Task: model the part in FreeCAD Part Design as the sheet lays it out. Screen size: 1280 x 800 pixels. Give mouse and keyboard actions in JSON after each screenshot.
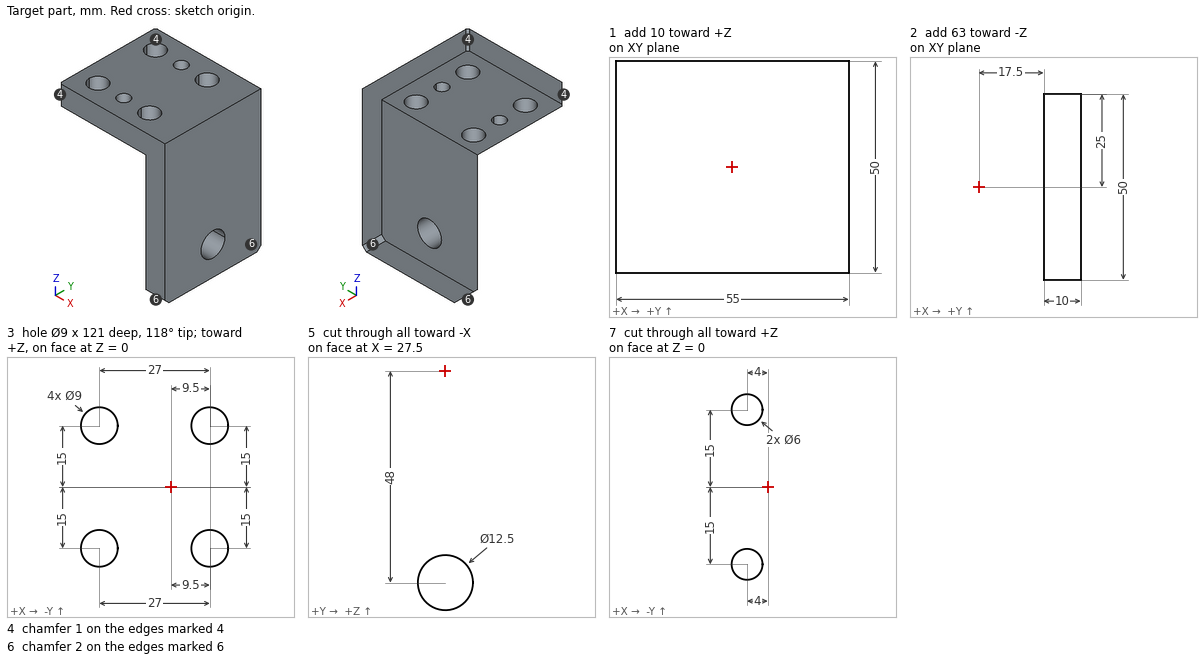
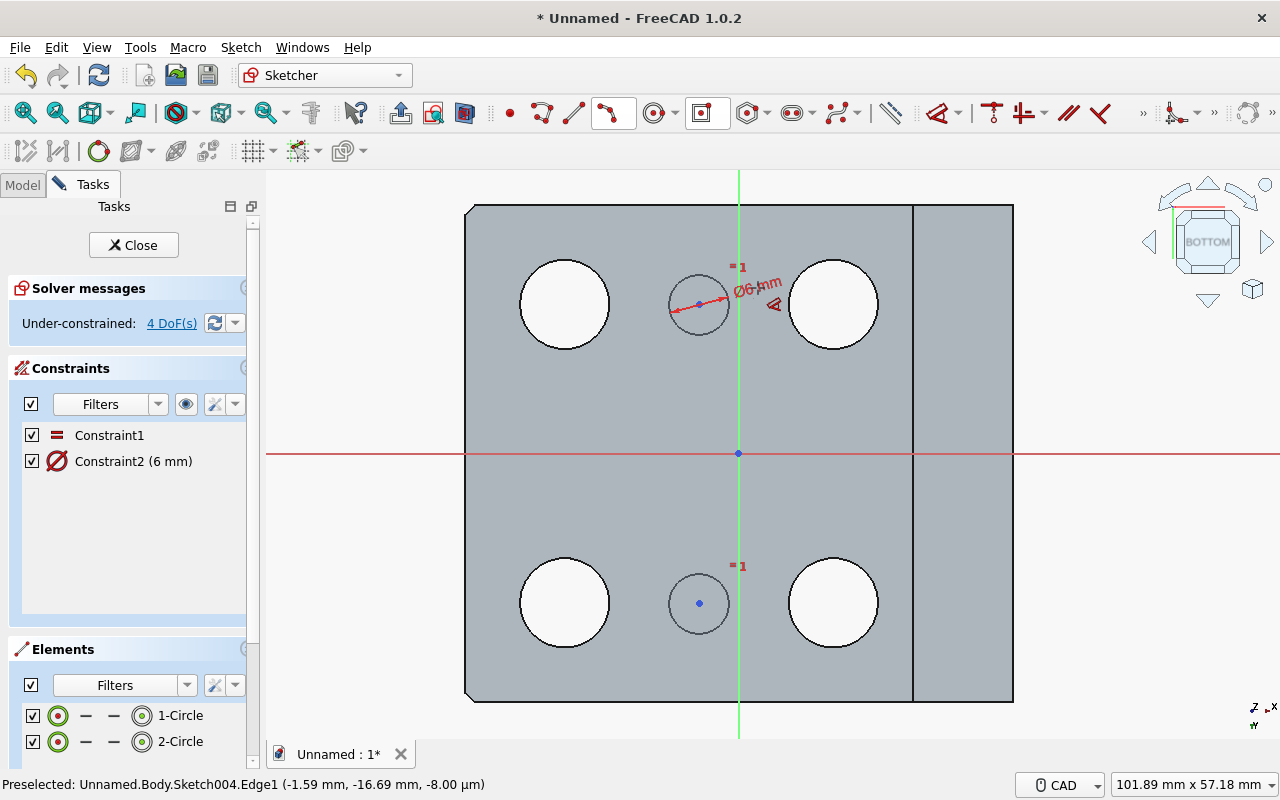
{"action": "left_click", "coordinate": [699, 305]}
{"action": "left_click", "coordinate": [719, 488]}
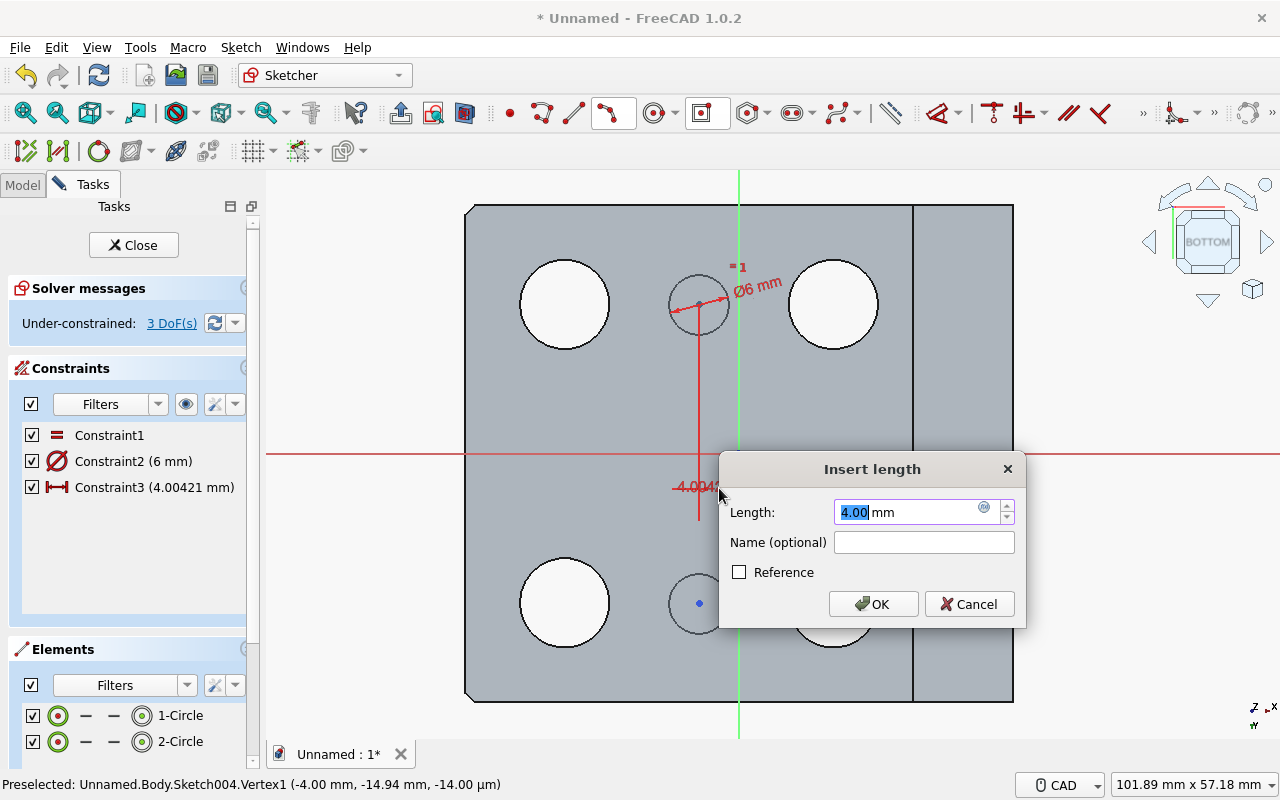
{"action": "type", "text": "4"}
{"action": "key", "text": "Return"}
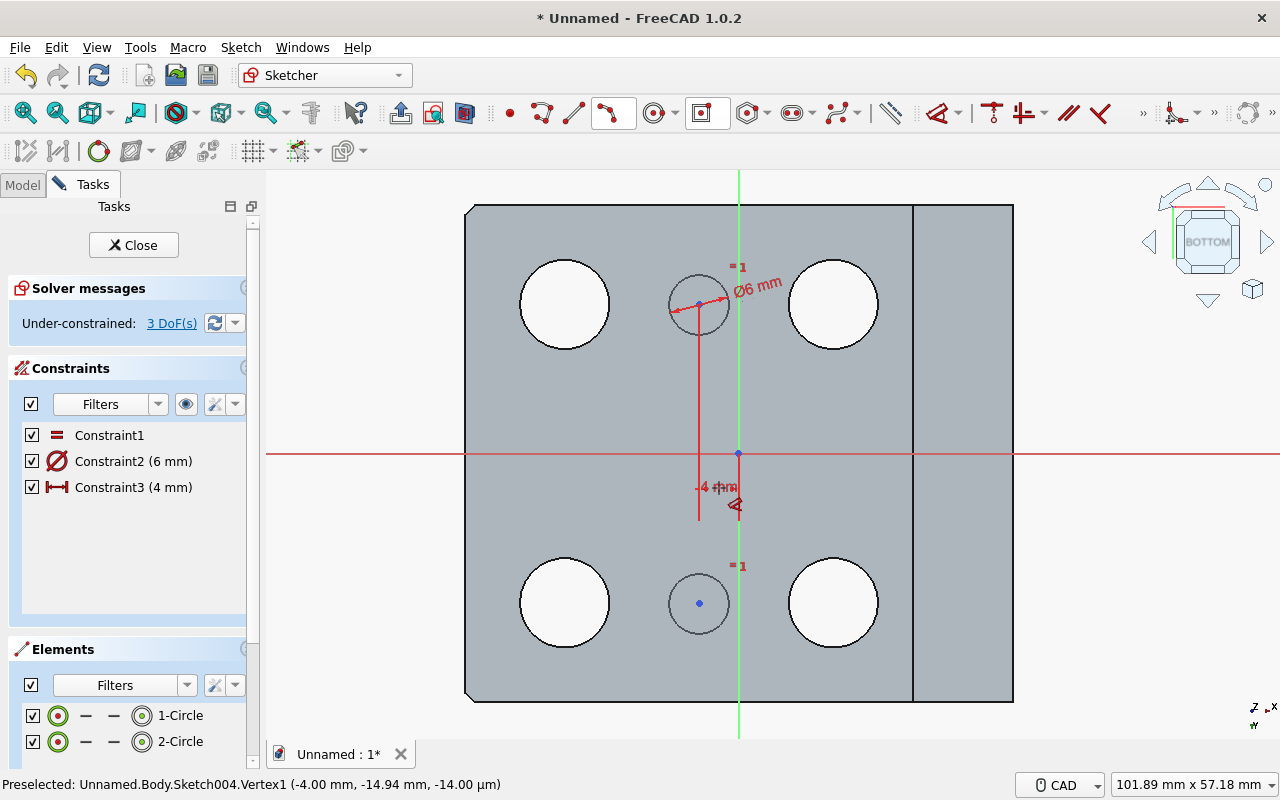
{"action": "left_click", "coordinate": [699, 604]}
{"action": "left_click", "coordinate": [719, 420]}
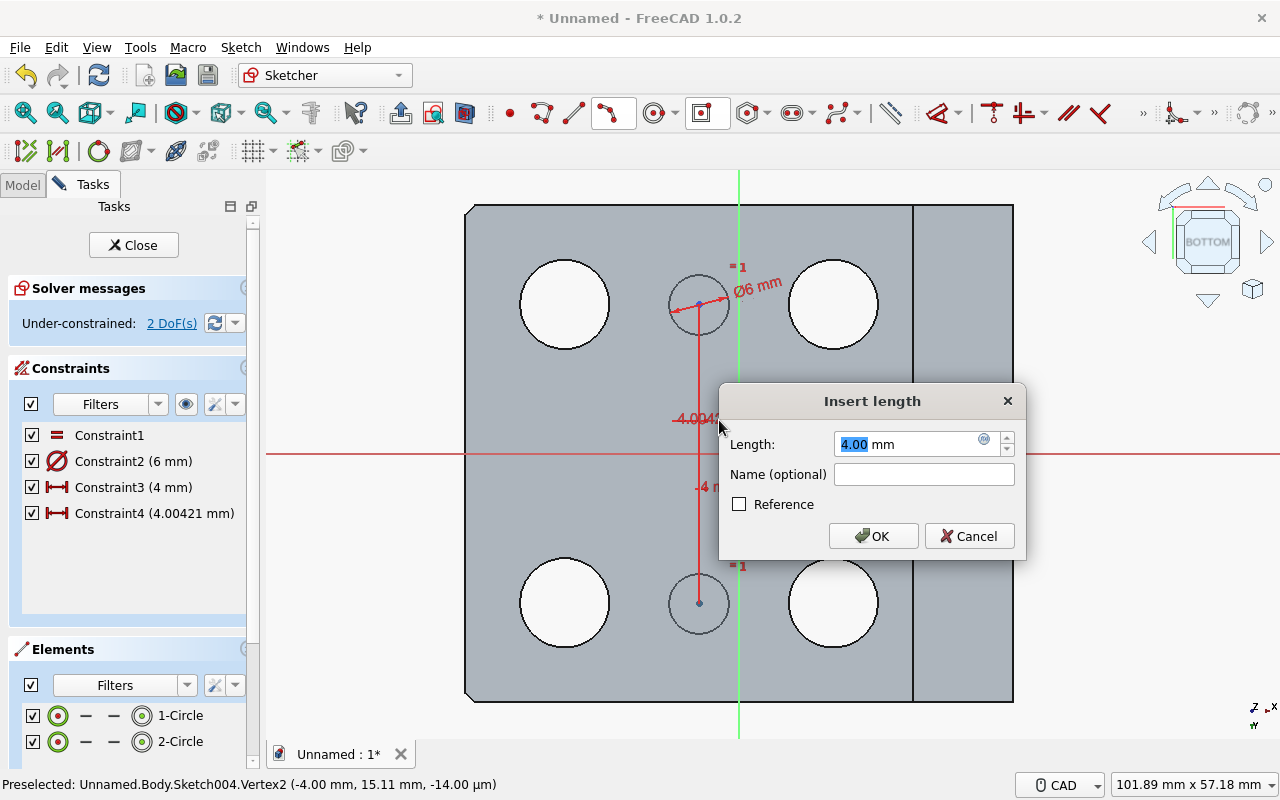
{"action": "type", "text": "4"}
{"action": "key", "text": "Return"}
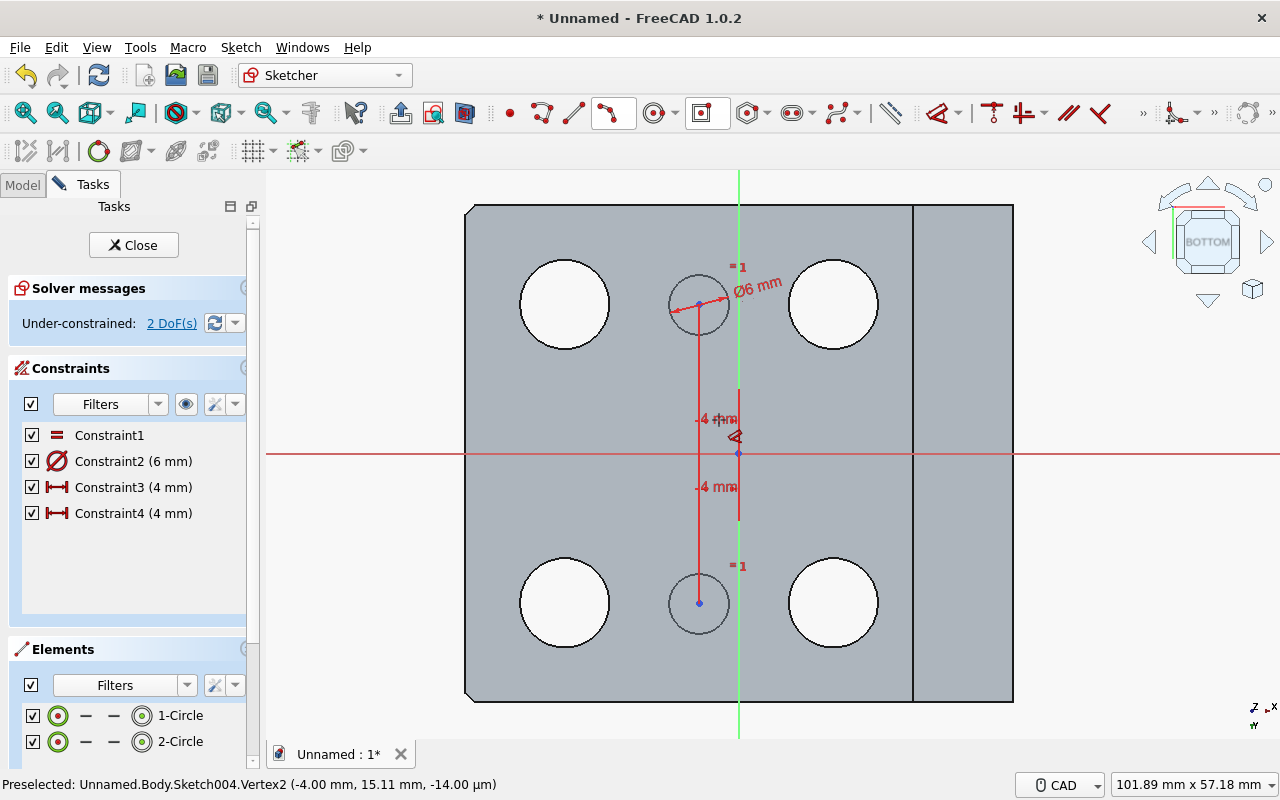
{"action": "left_click", "coordinate": [699, 305]}
{"action": "left_click", "coordinate": [773, 379]}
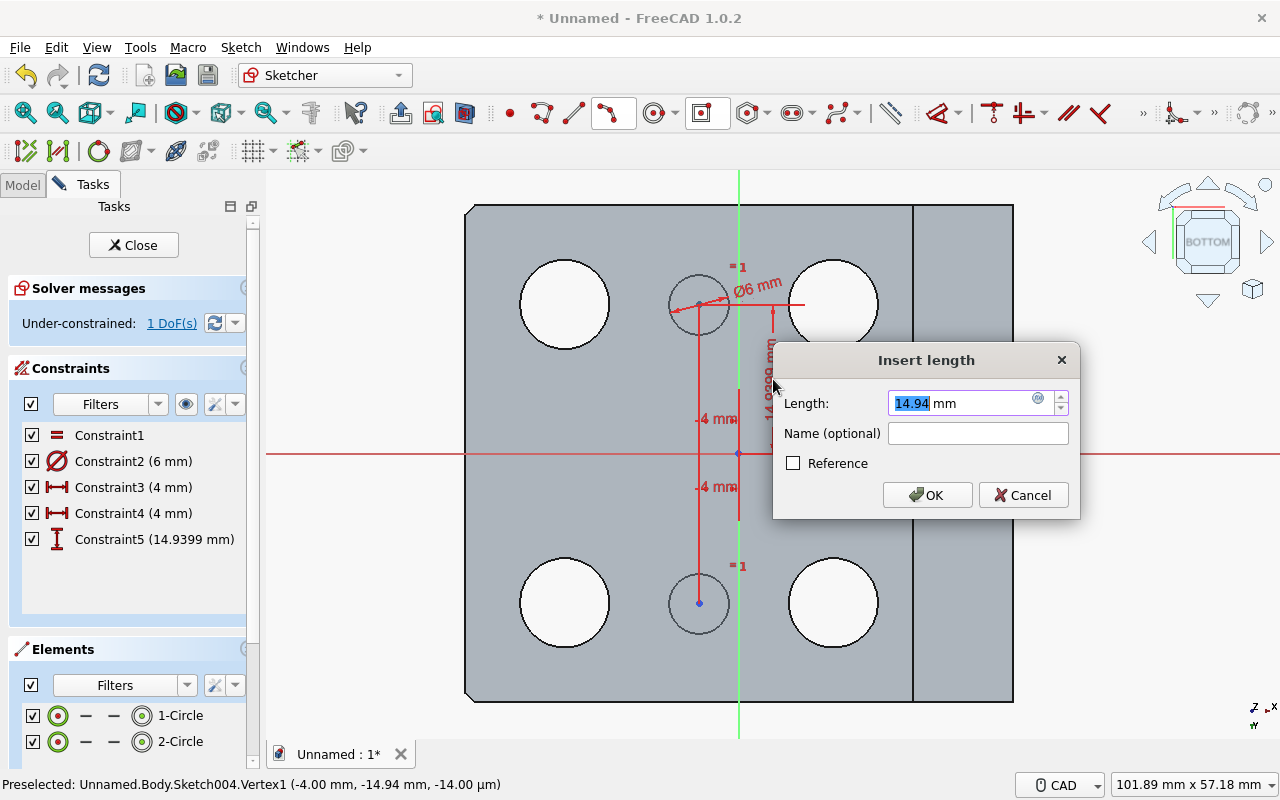
{"action": "type", "text": "15"}
{"action": "key", "text": "Return"}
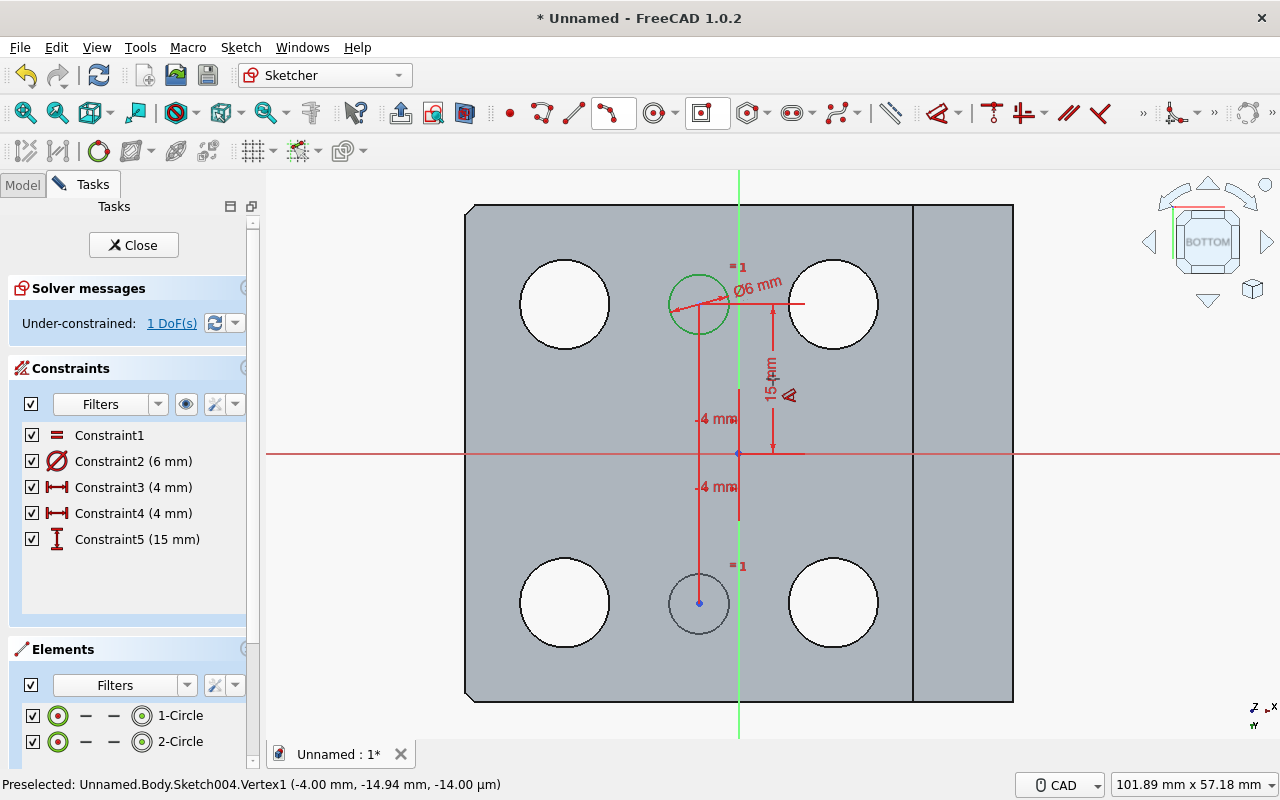
{"action": "left_click", "coordinate": [699, 604]}
{"action": "left_click", "coordinate": [773, 529]}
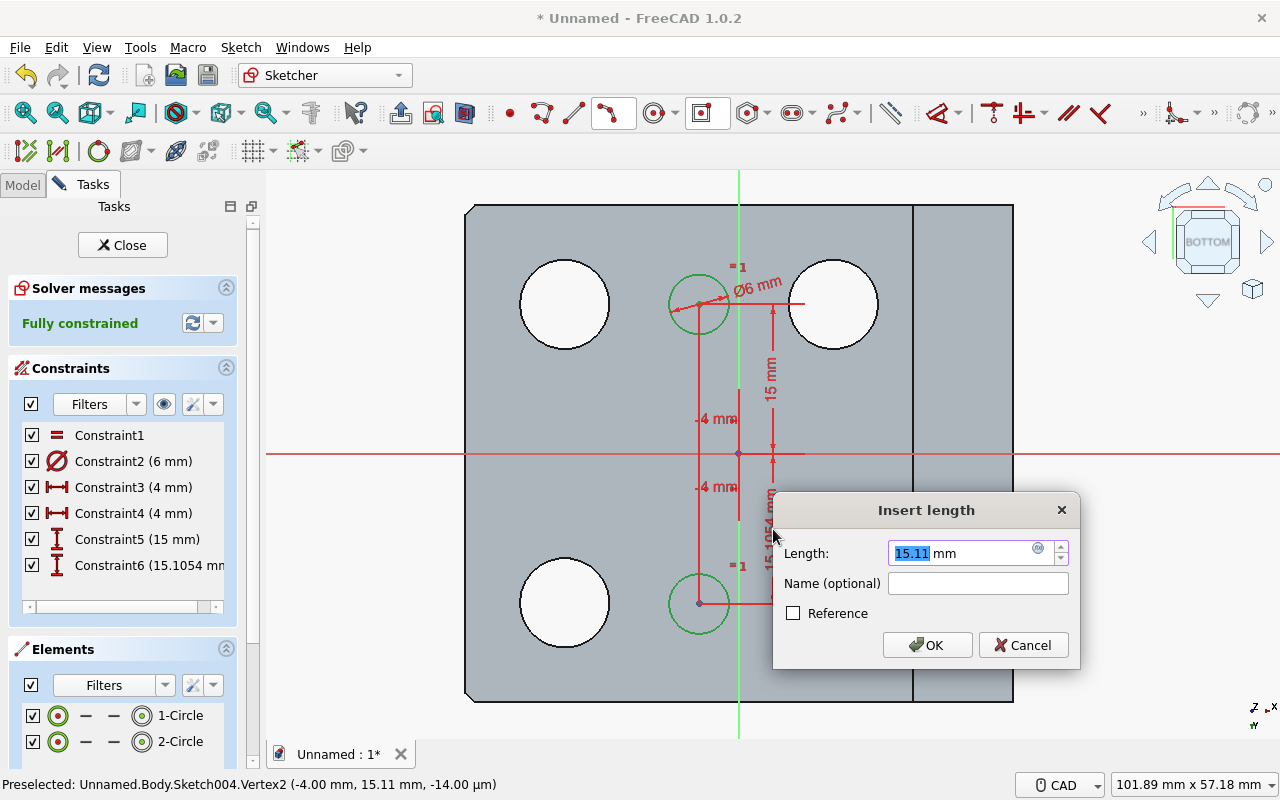
{"action": "type", "text": "15"}
{"action": "key", "text": "Return"}
{"action": "key", "text": "Escape"}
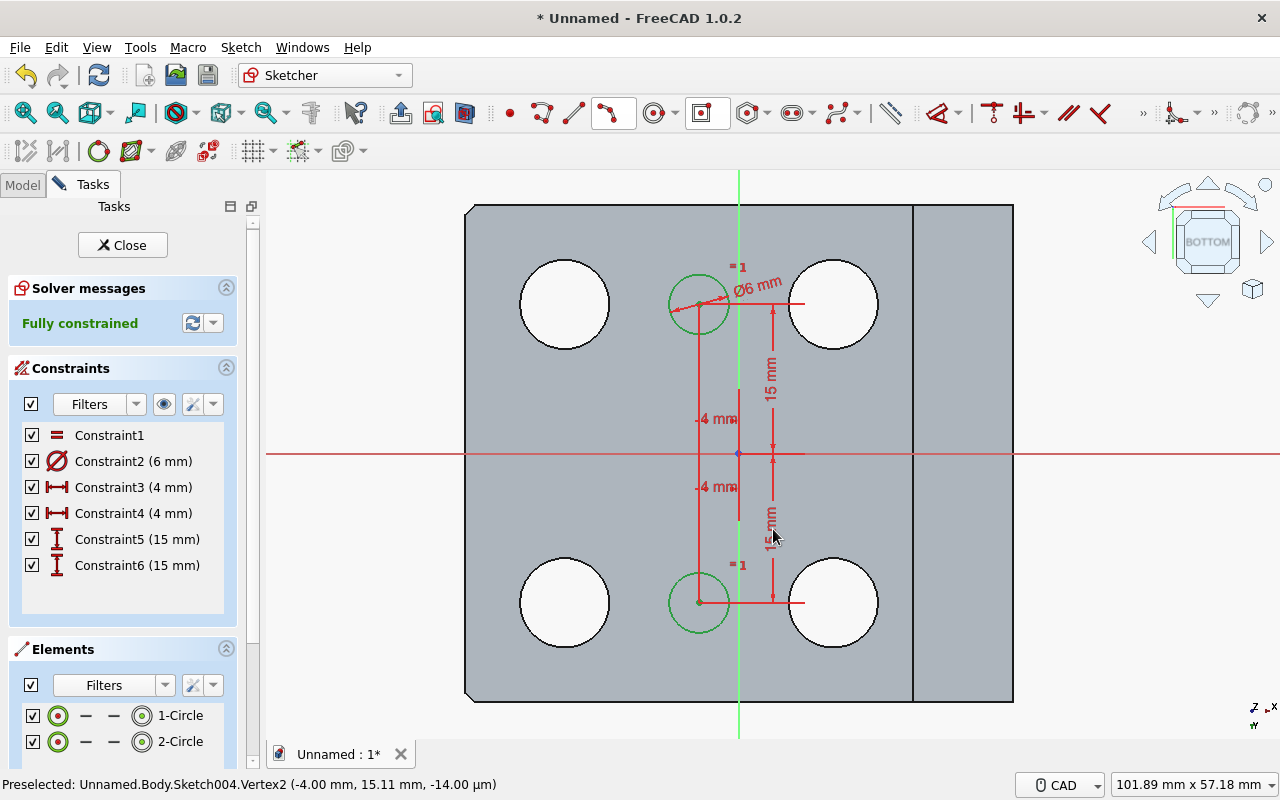
{"action": "left_click", "coordinate": [123, 245]}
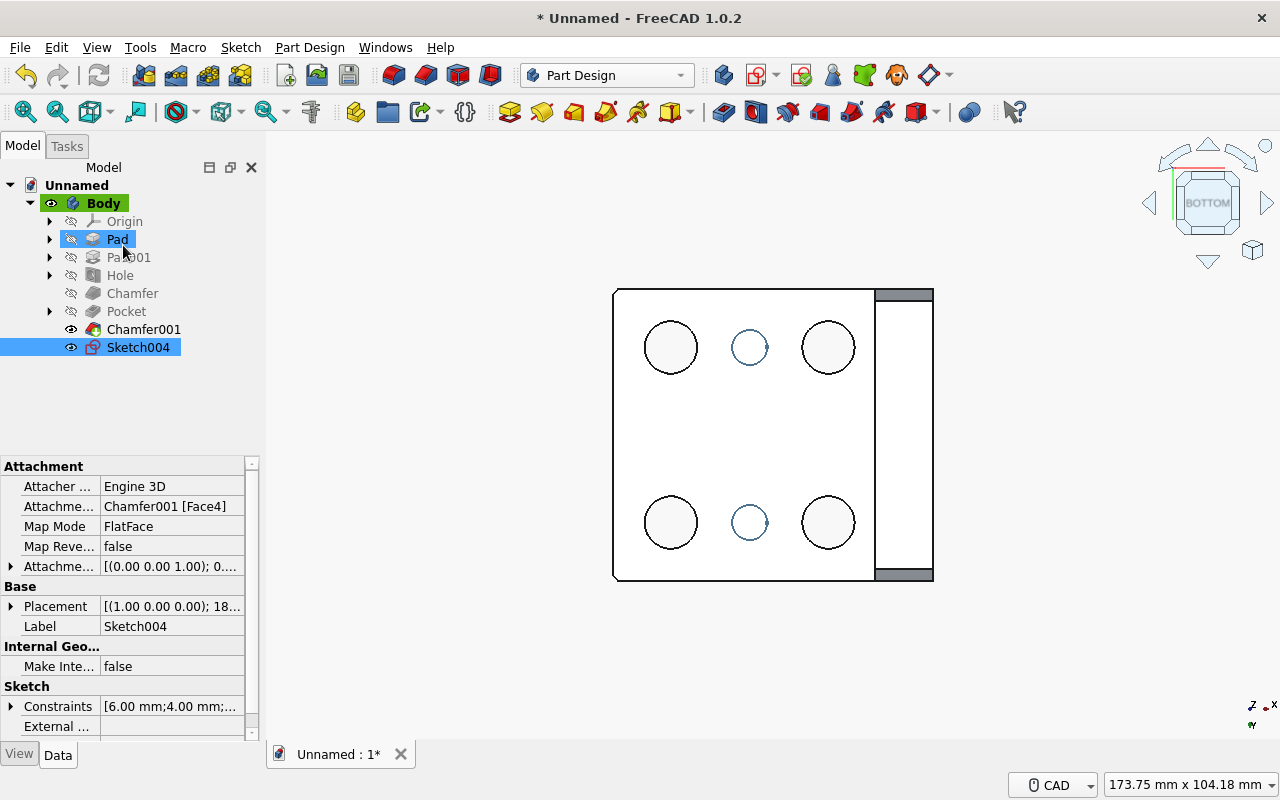
{"action": "left_click", "coordinate": [724, 112]}